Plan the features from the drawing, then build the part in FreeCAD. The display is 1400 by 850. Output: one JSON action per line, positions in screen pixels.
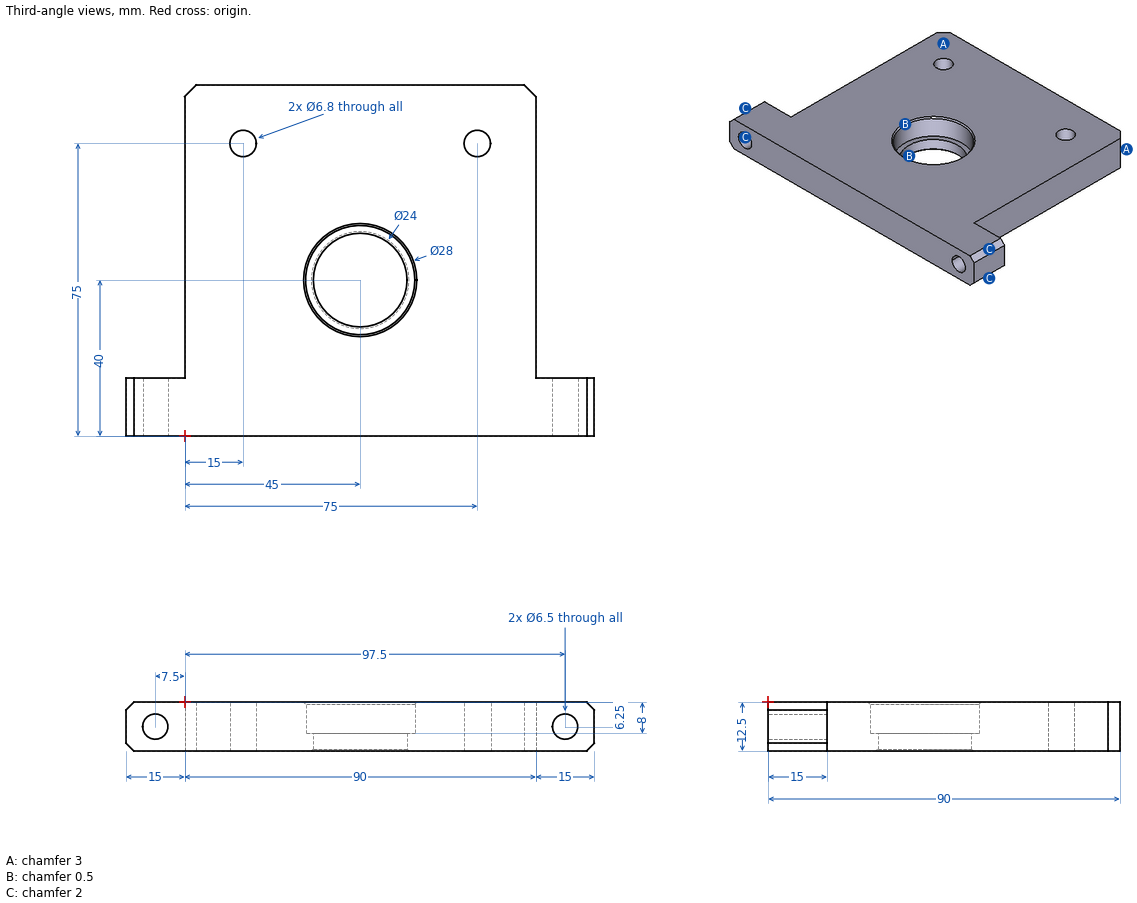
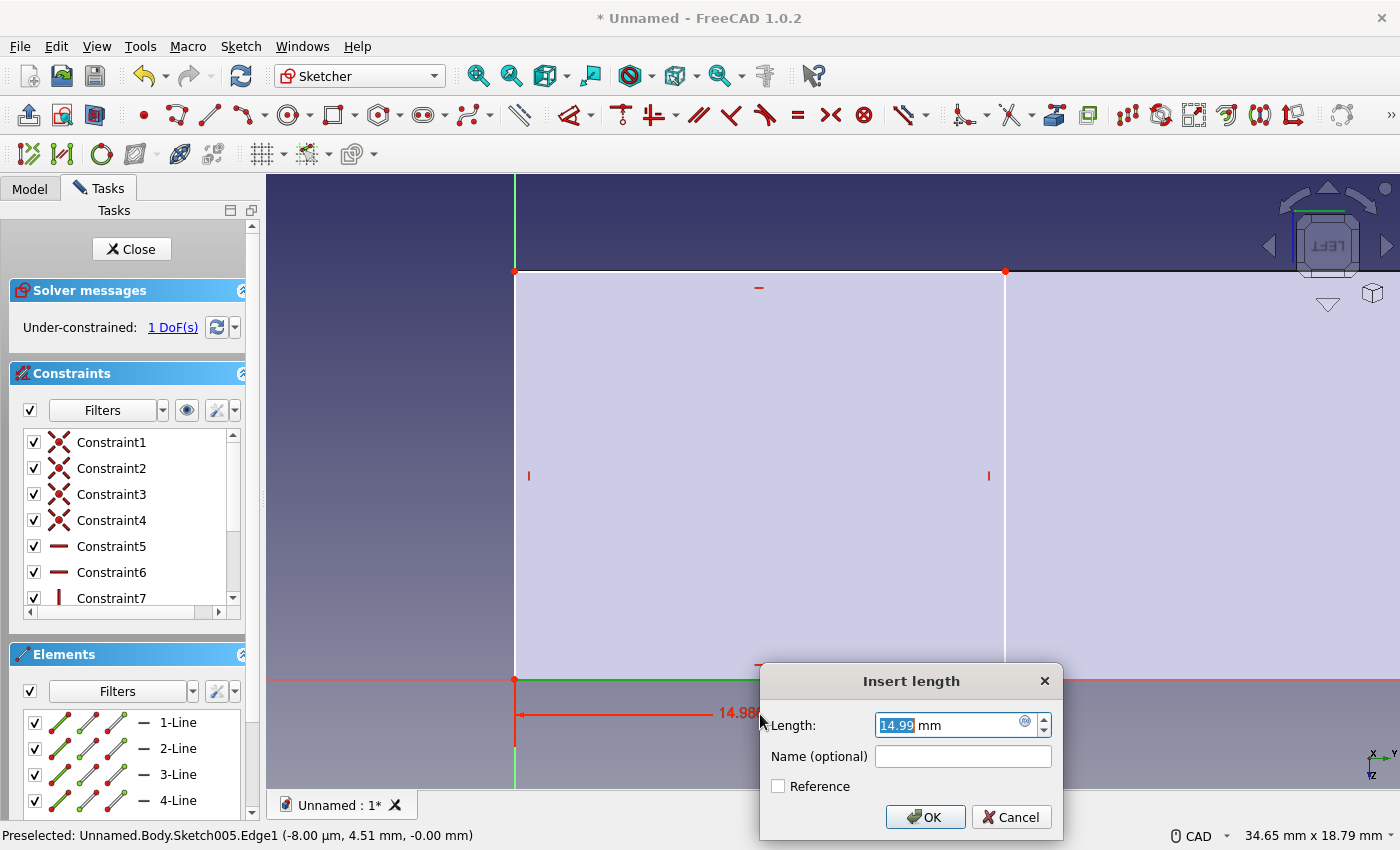
{"action": "type", "text": "15"}
{"action": "key", "text": "Return"}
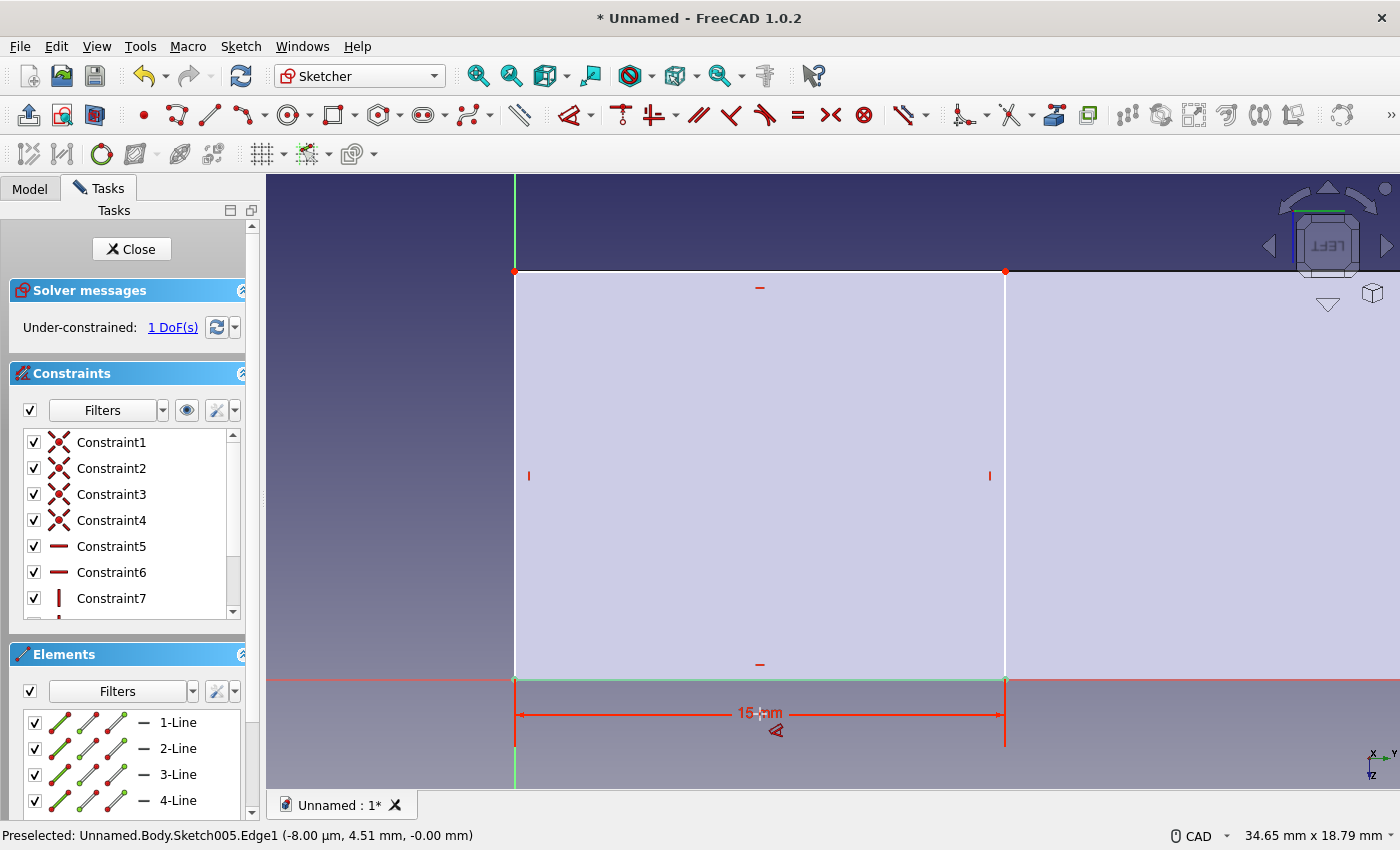
{"action": "left_click", "coordinate": [1005, 557]}
{"action": "left_click", "coordinate": [1039, 476]}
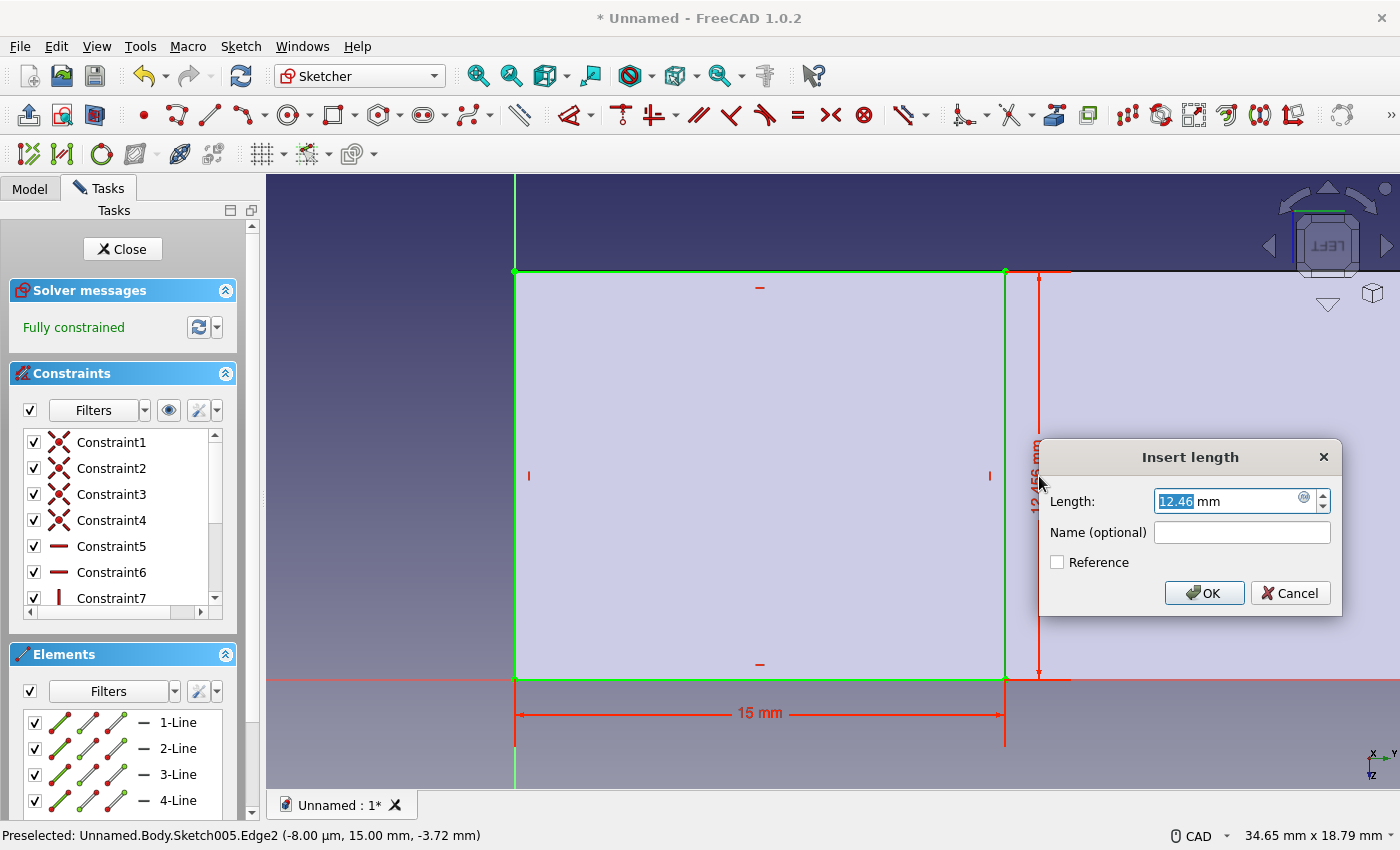
{"action": "type", "text": "12.5"}
{"action": "key", "text": "Return"}
{"action": "key", "text": "Escape"}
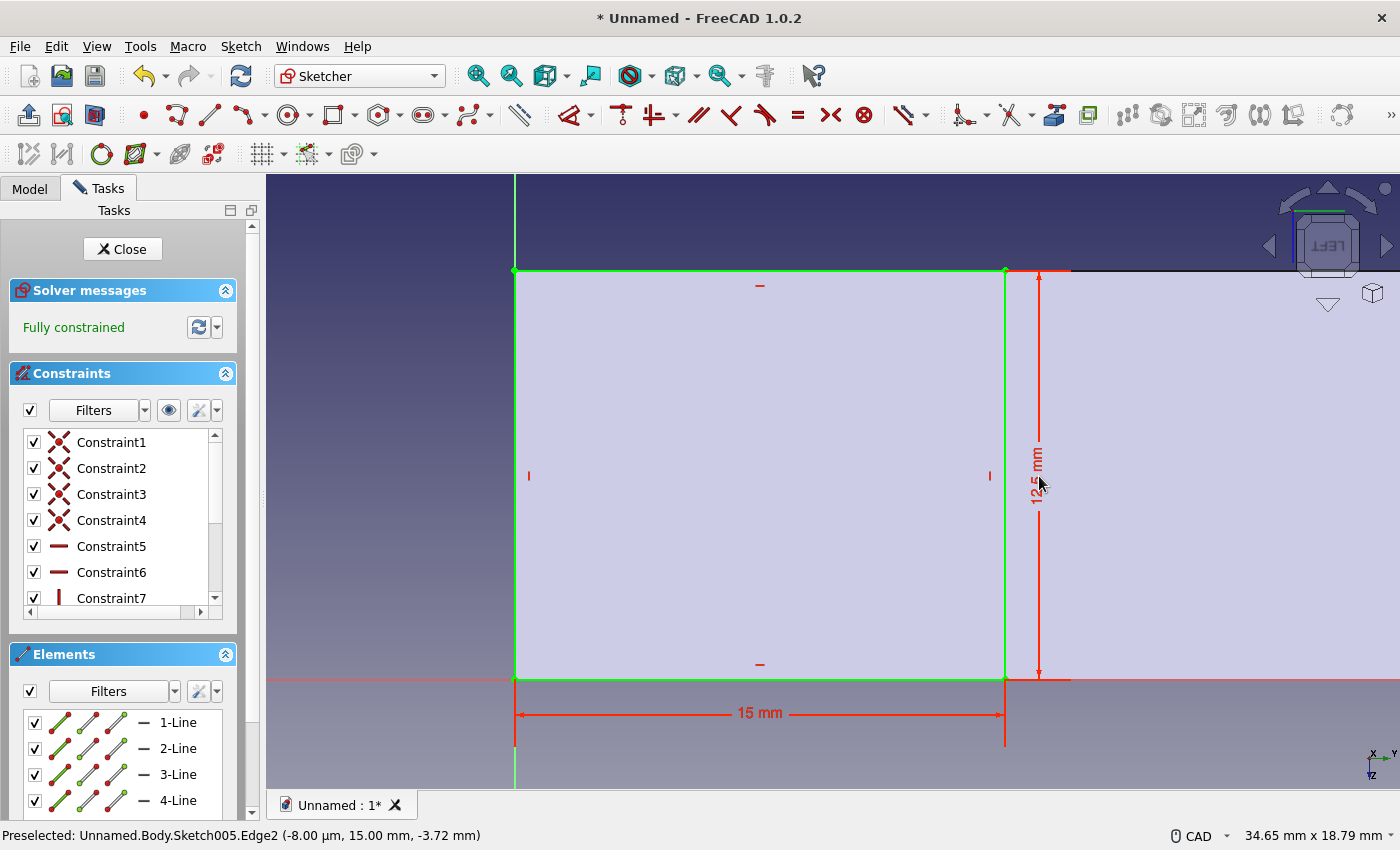
{"action": "left_click", "coordinate": [123, 249]}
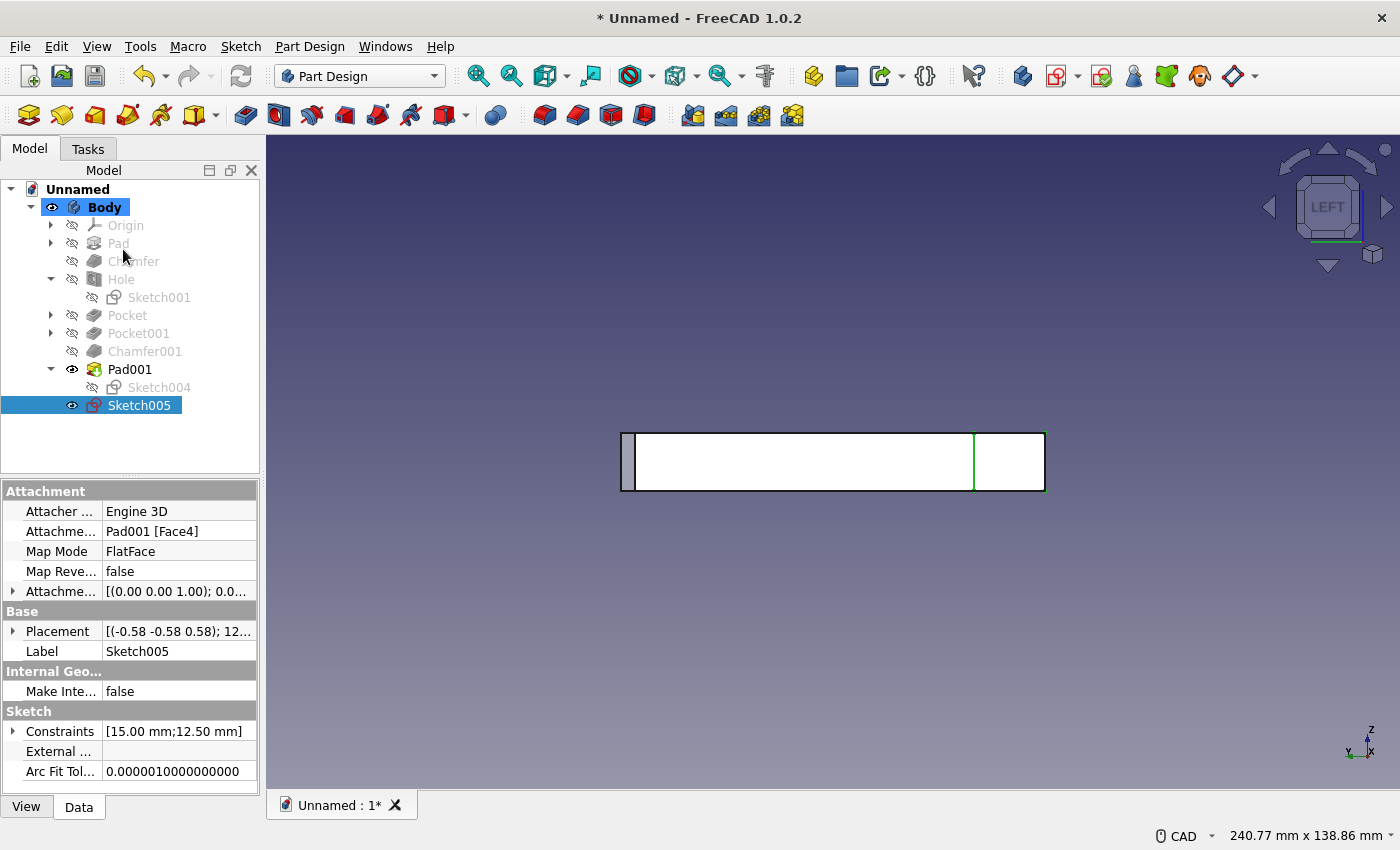
{"action": "left_click", "coordinate": [29, 116]}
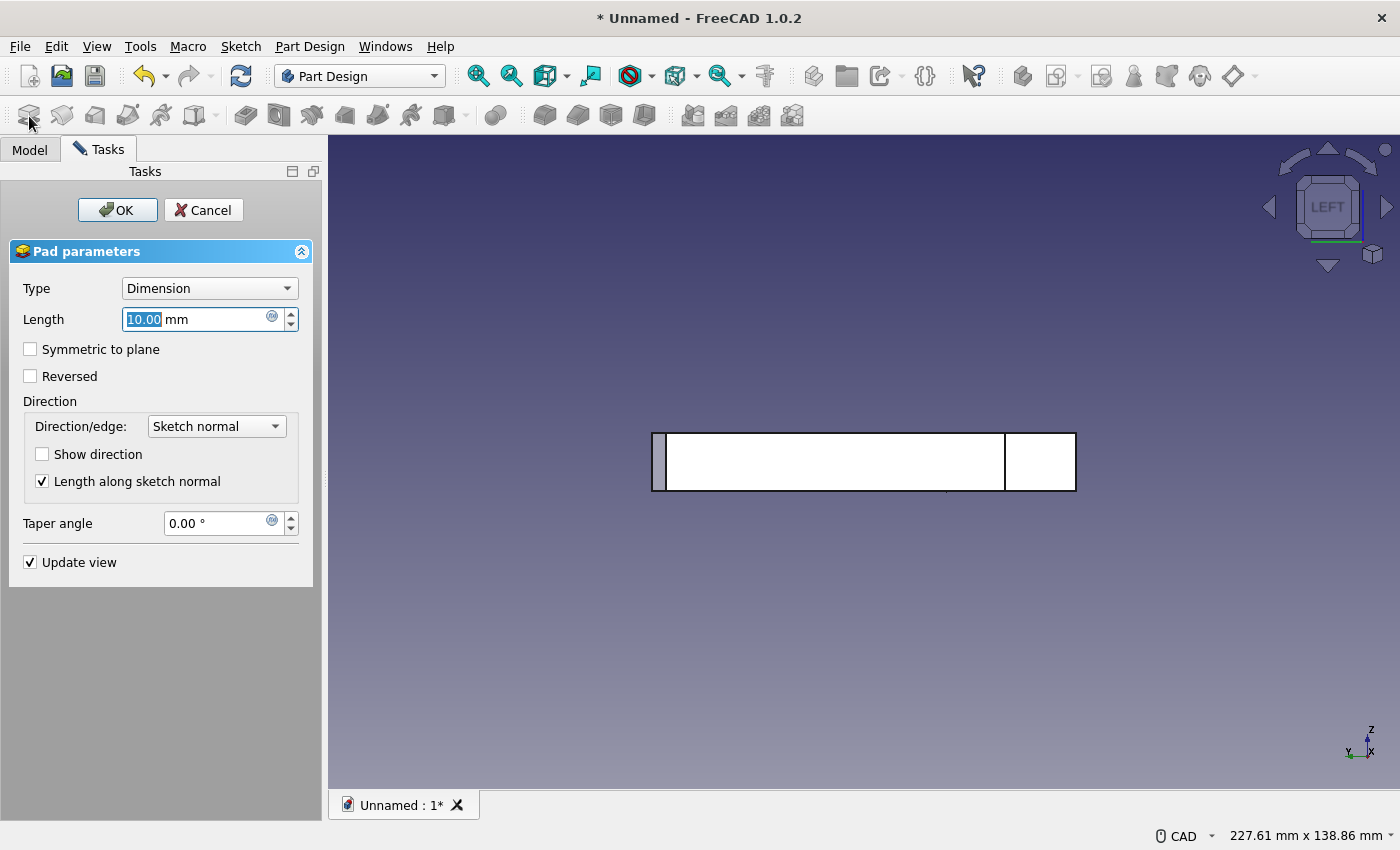
{"action": "type", "text": "15"}
{"action": "key", "text": "Tab"}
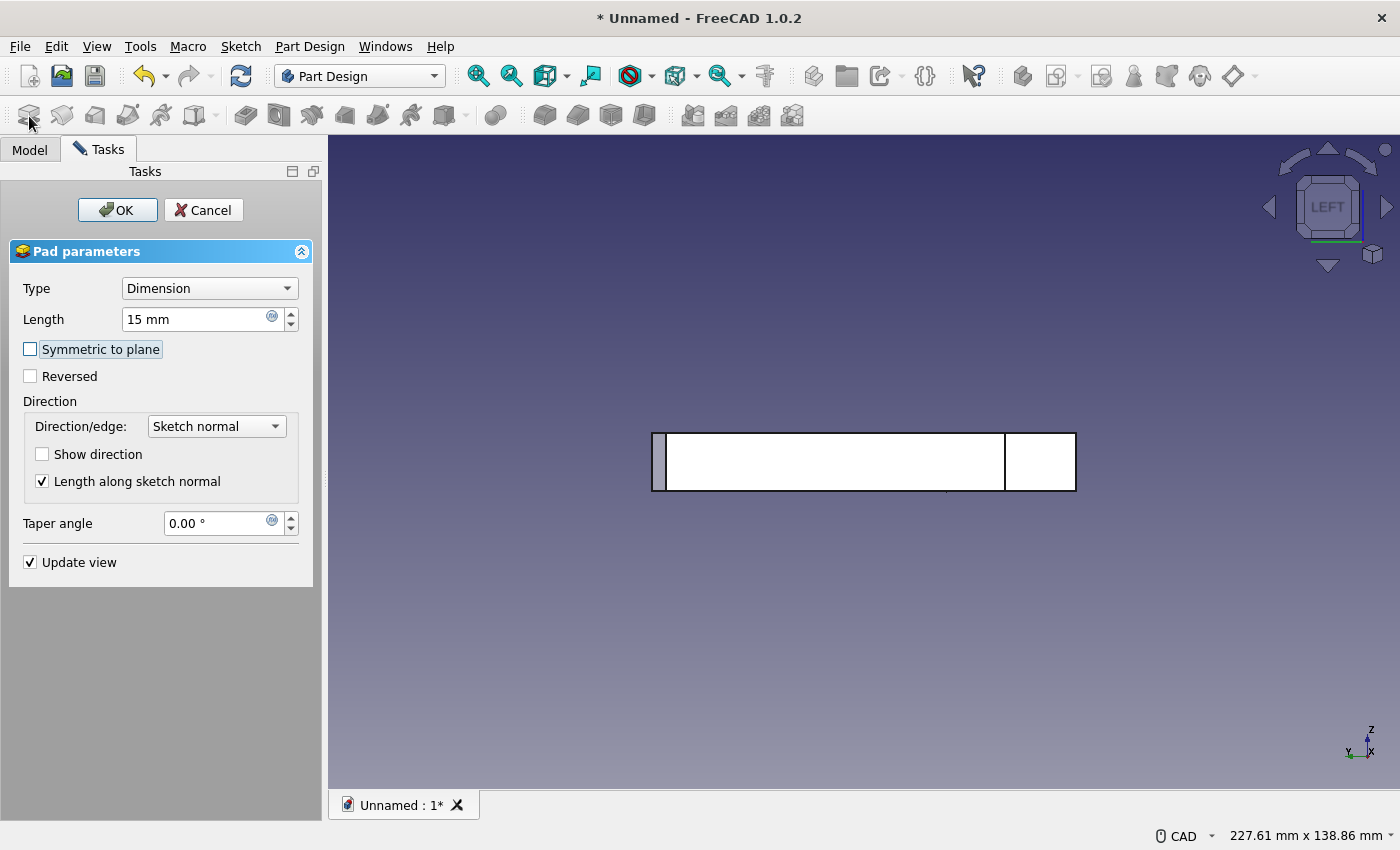
{"action": "left_click", "coordinate": [118, 210]}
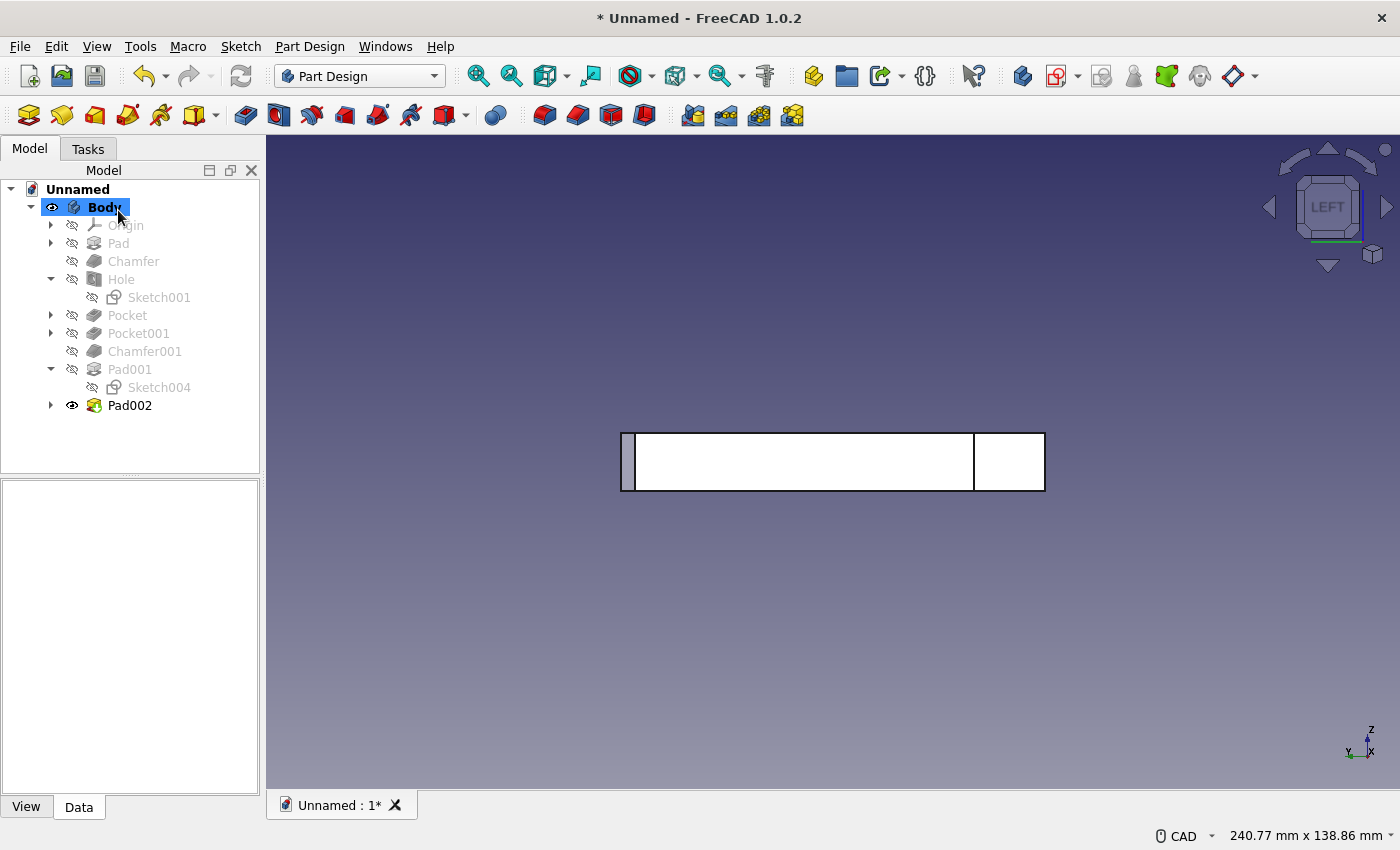
{"action": "left_click", "coordinate": [479, 76]}